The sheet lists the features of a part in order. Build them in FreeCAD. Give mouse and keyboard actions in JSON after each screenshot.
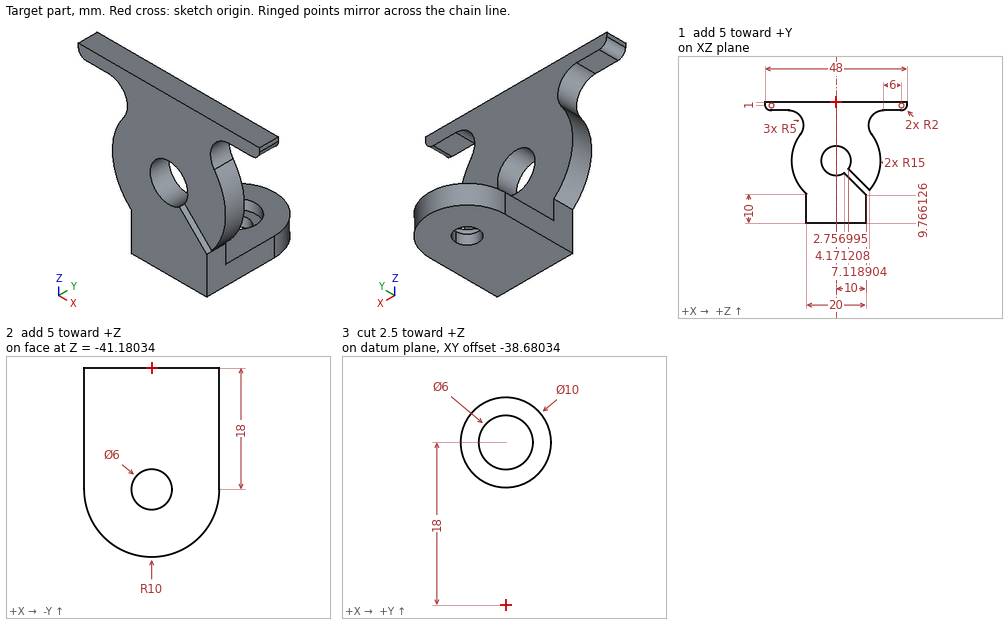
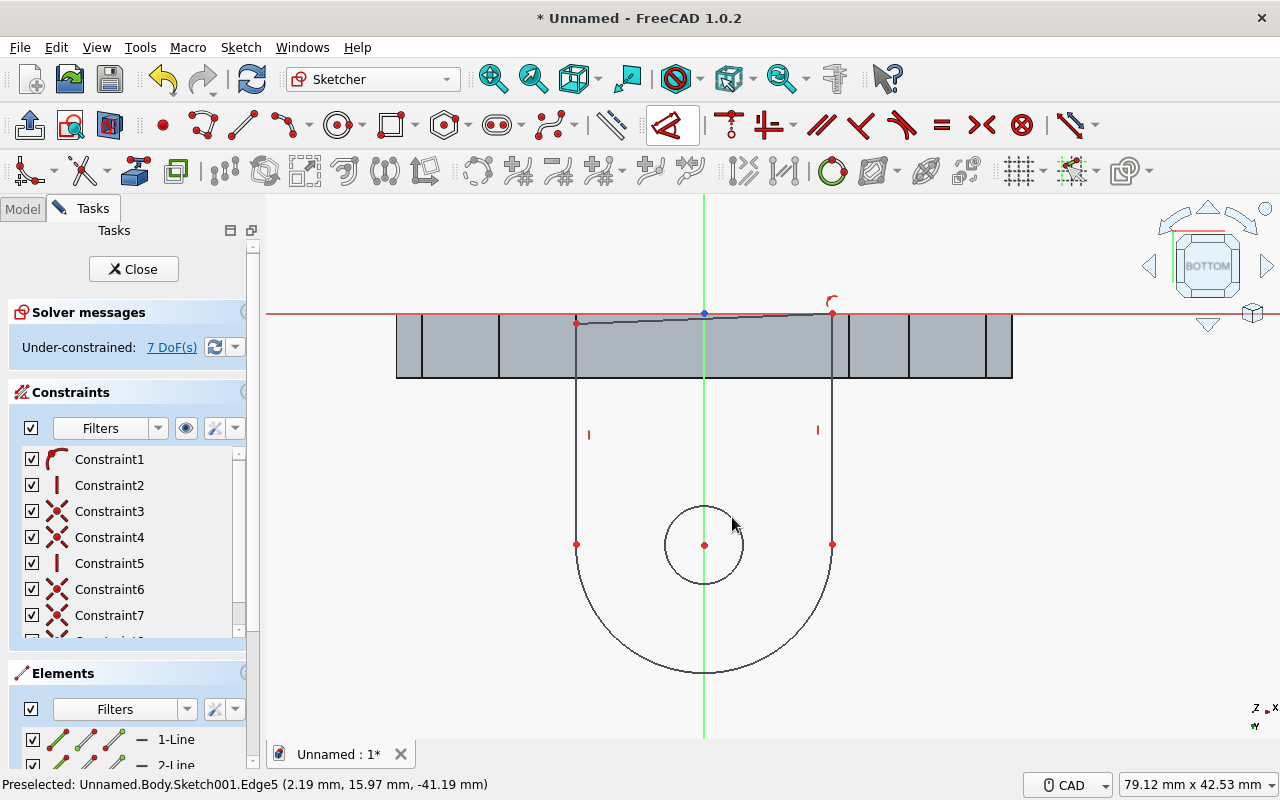
{"action": "left_click", "coordinate": [832, 476]}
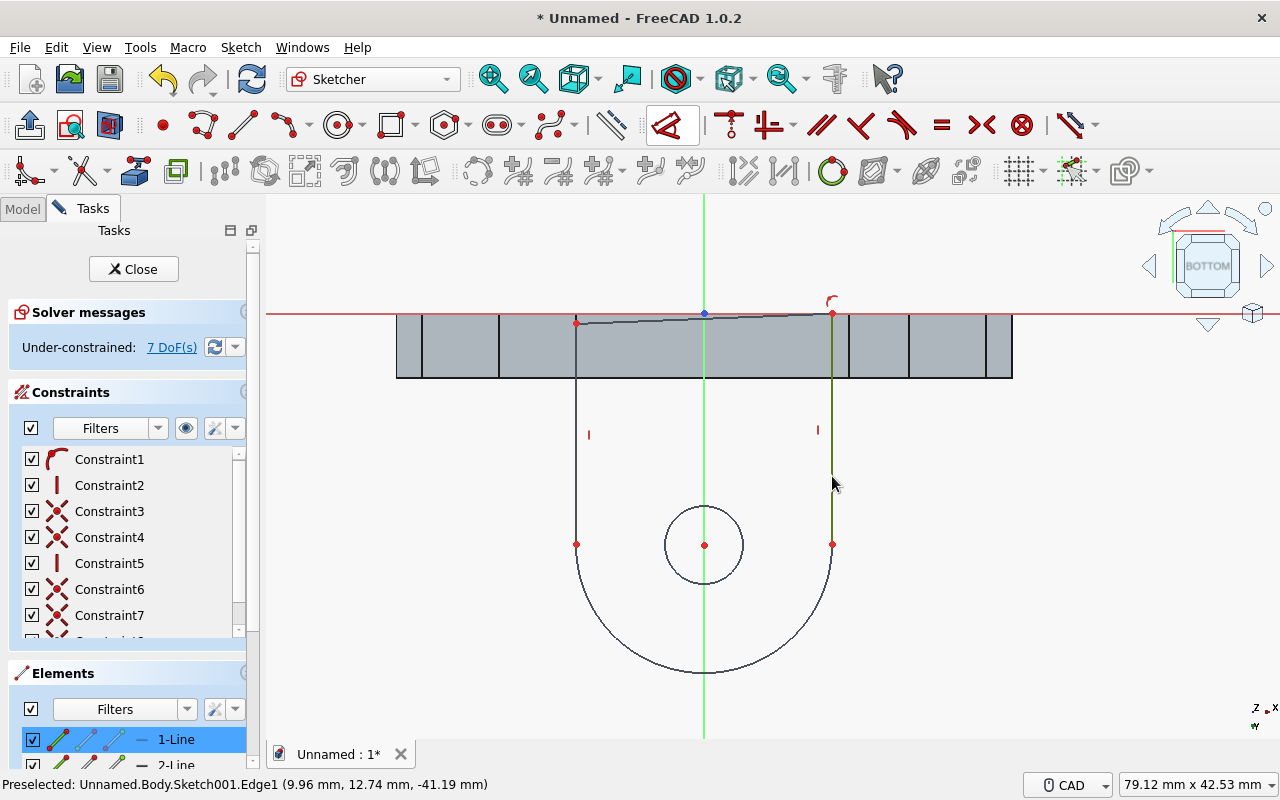
{"action": "left_click", "coordinate": [629, 649]}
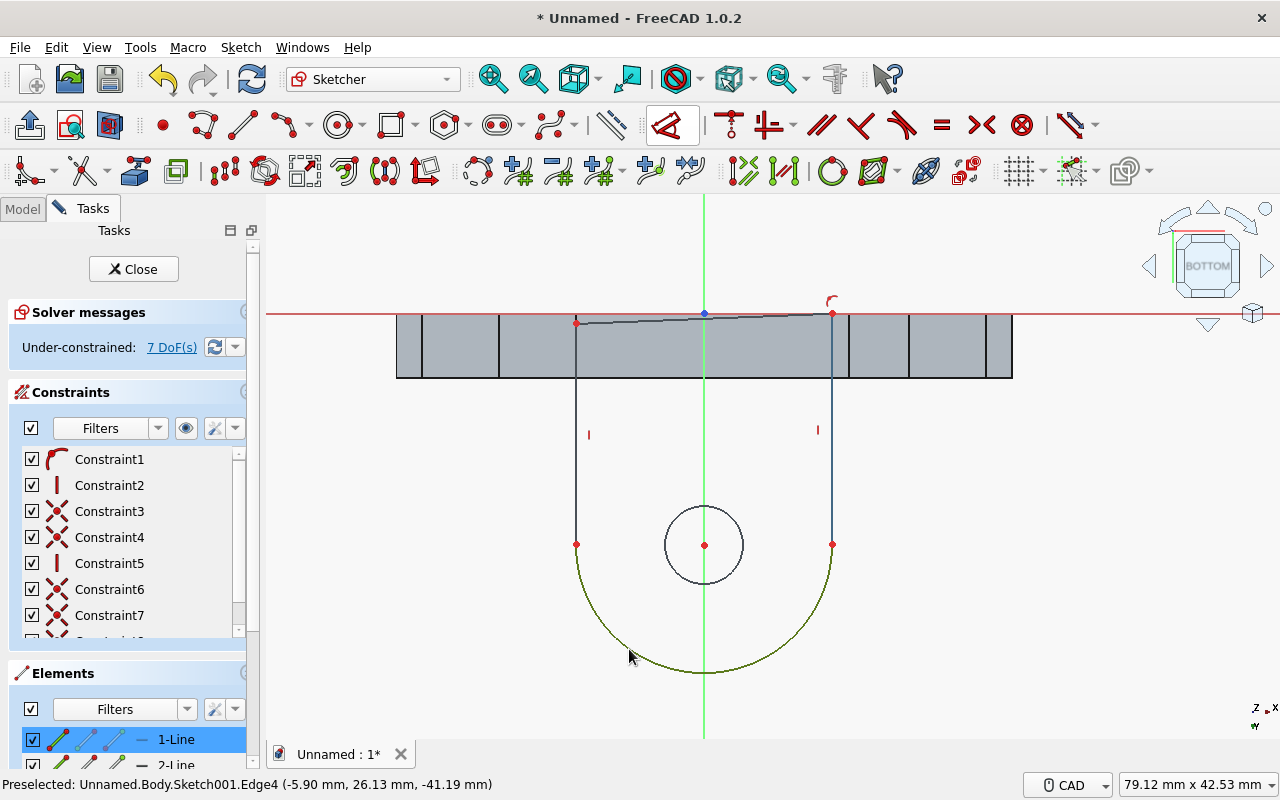
{"action": "key", "text": "t"}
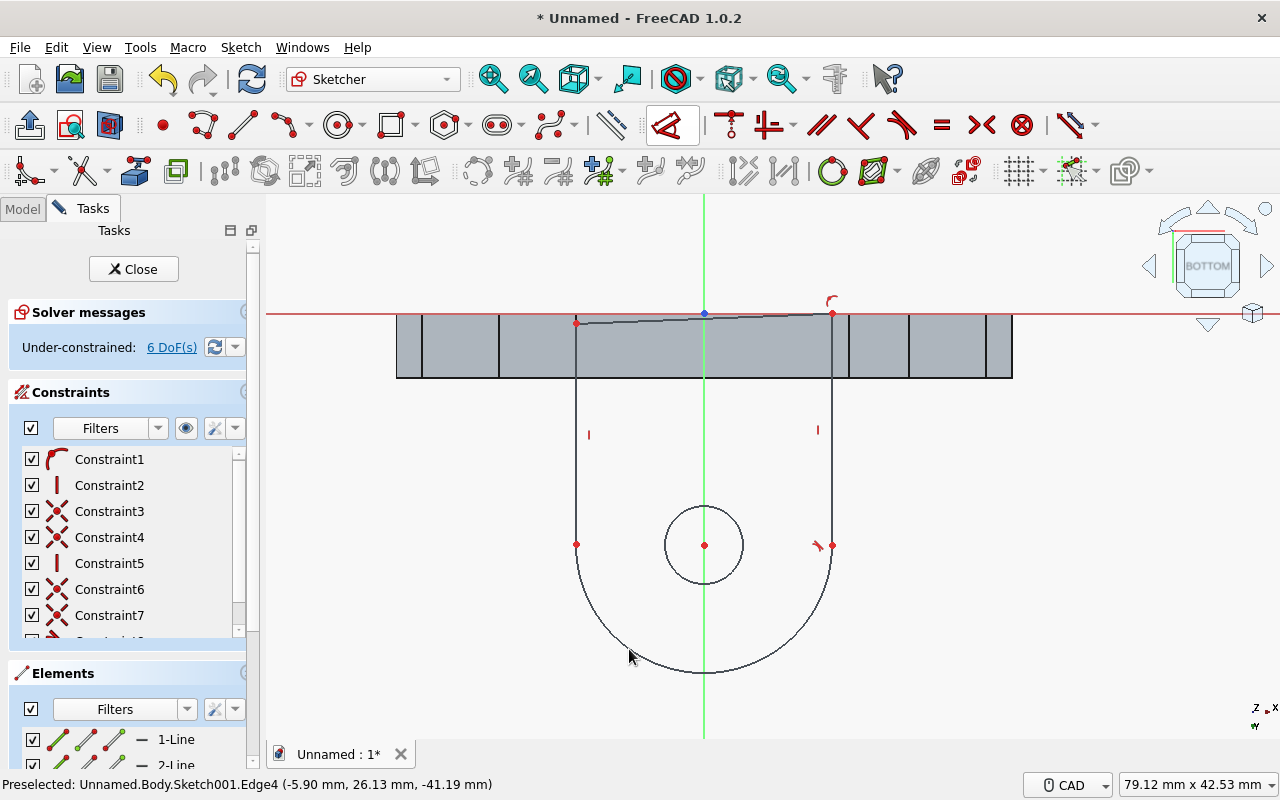
{"action": "left_click", "coordinate": [576, 390]}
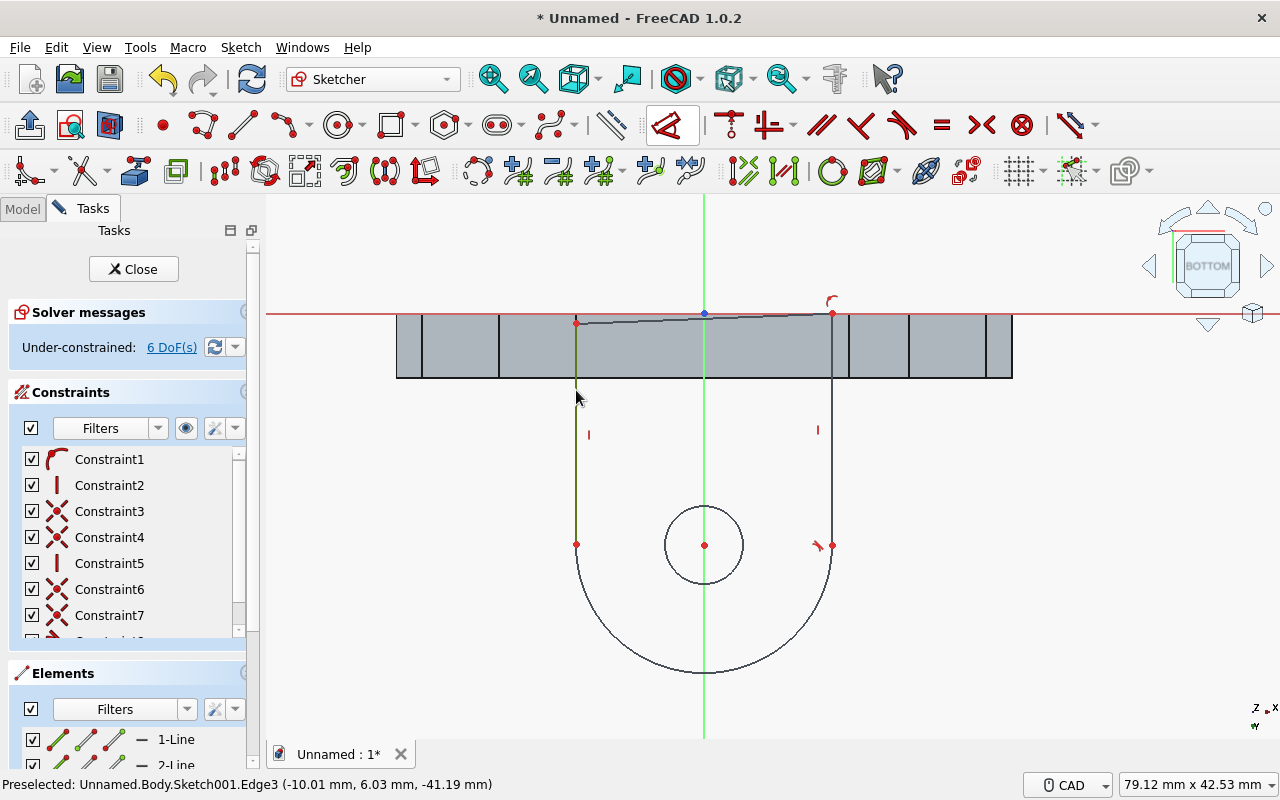
{"action": "left_click", "coordinate": [629, 649]}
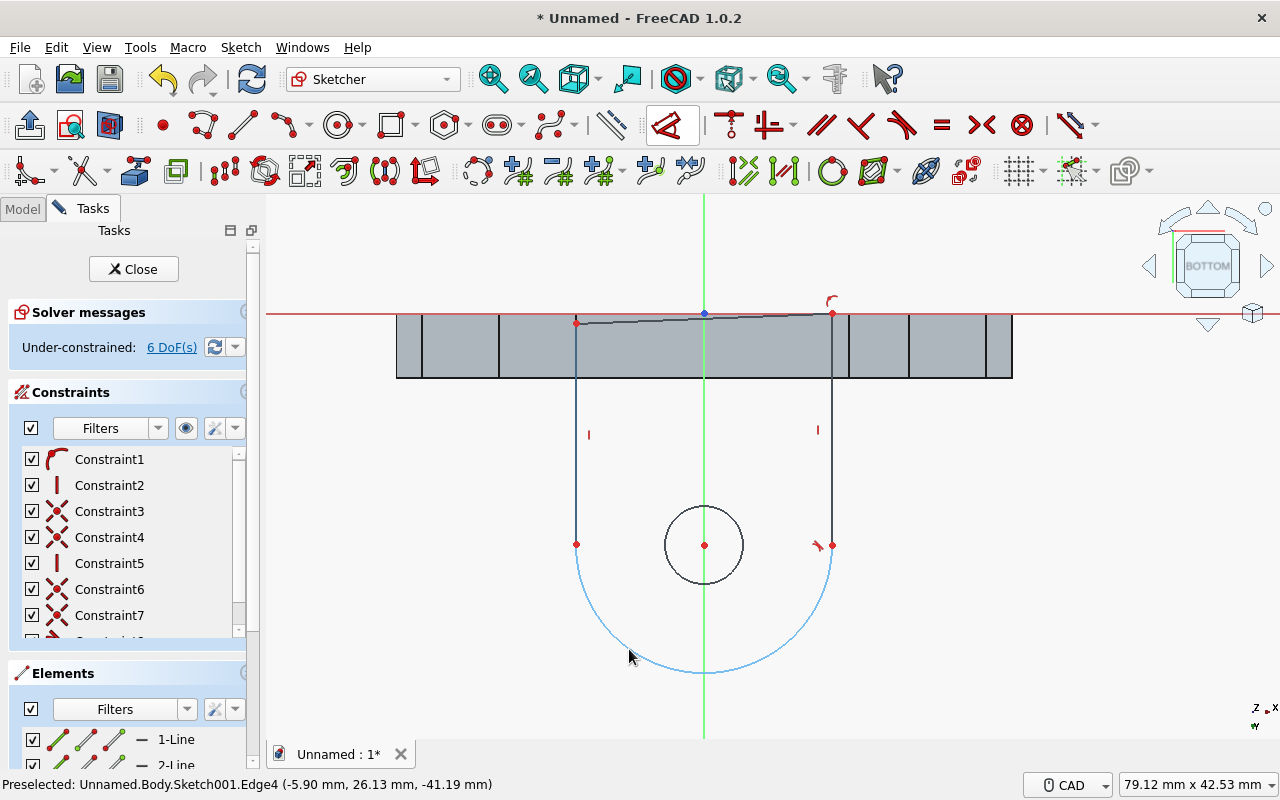
{"action": "key", "text": "t"}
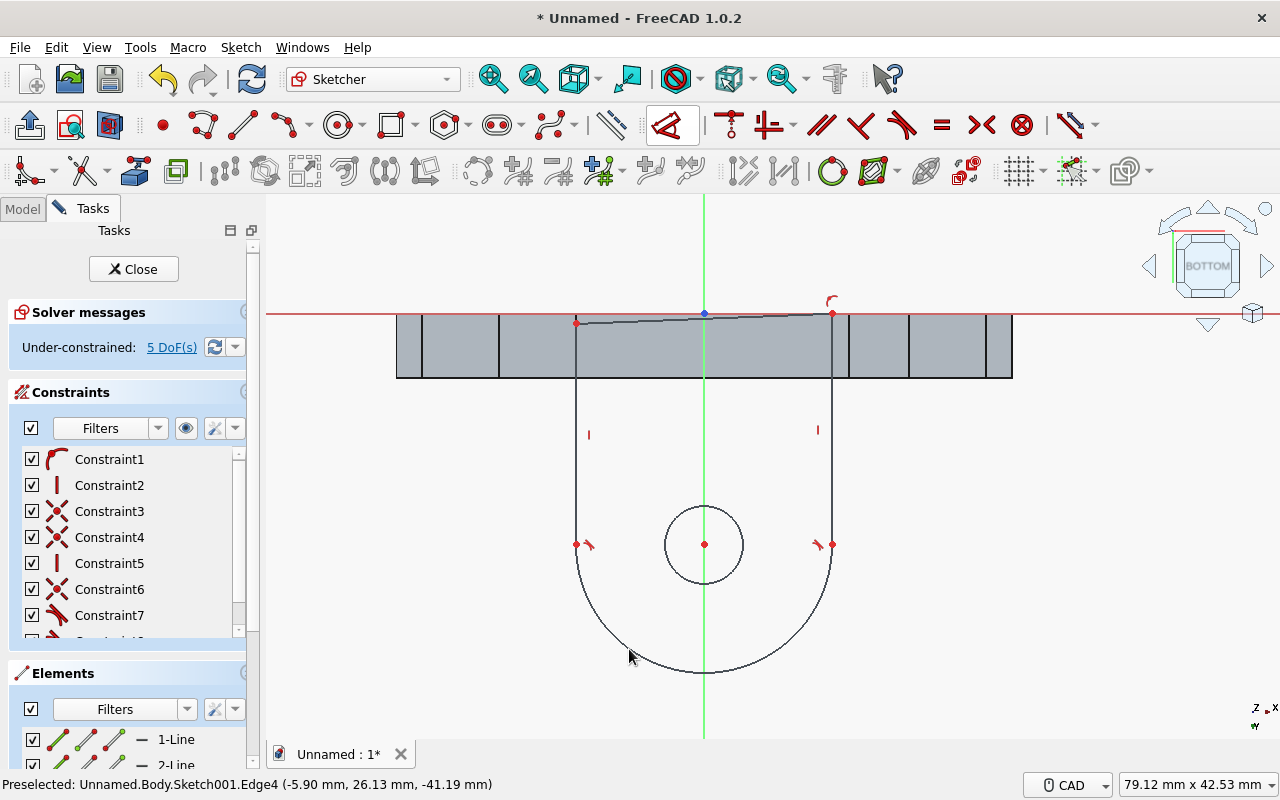
{"action": "left_click", "coordinate": [755, 317]}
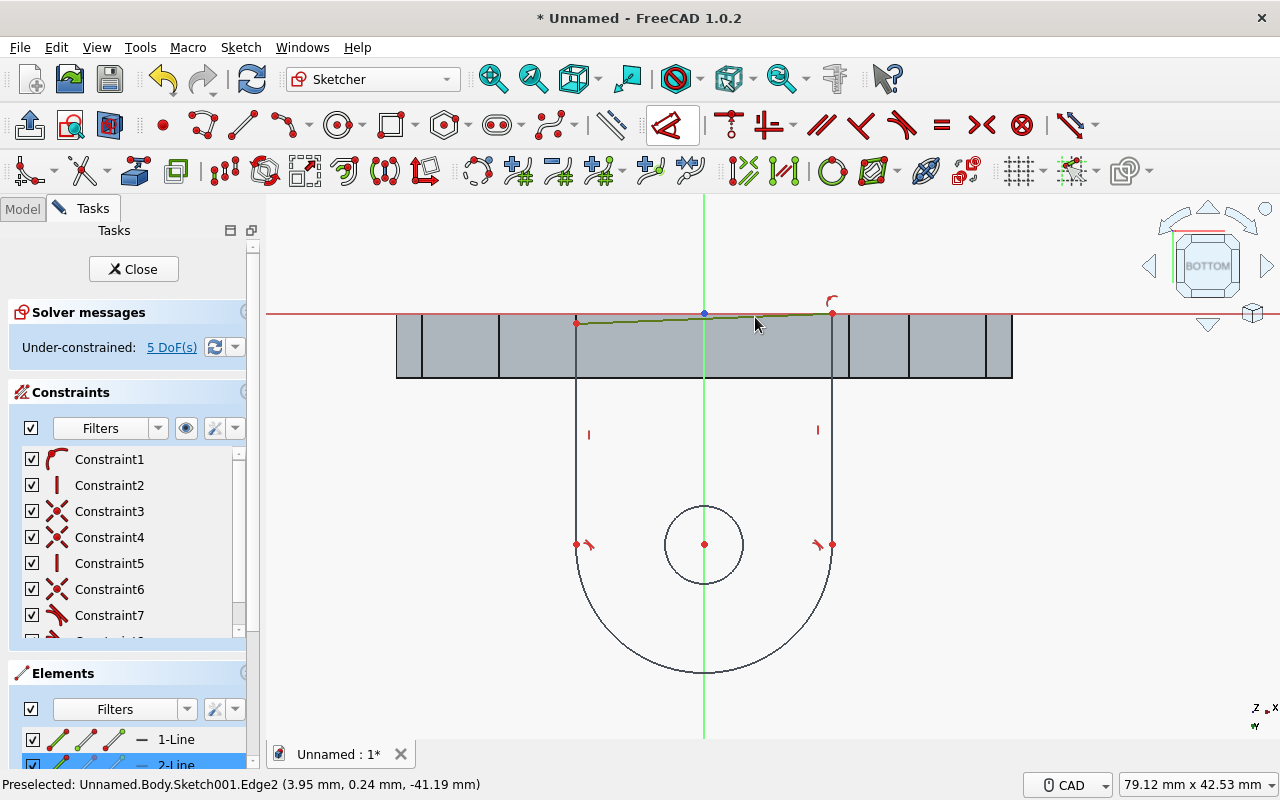
{"action": "left_click", "coordinate": [796, 126]}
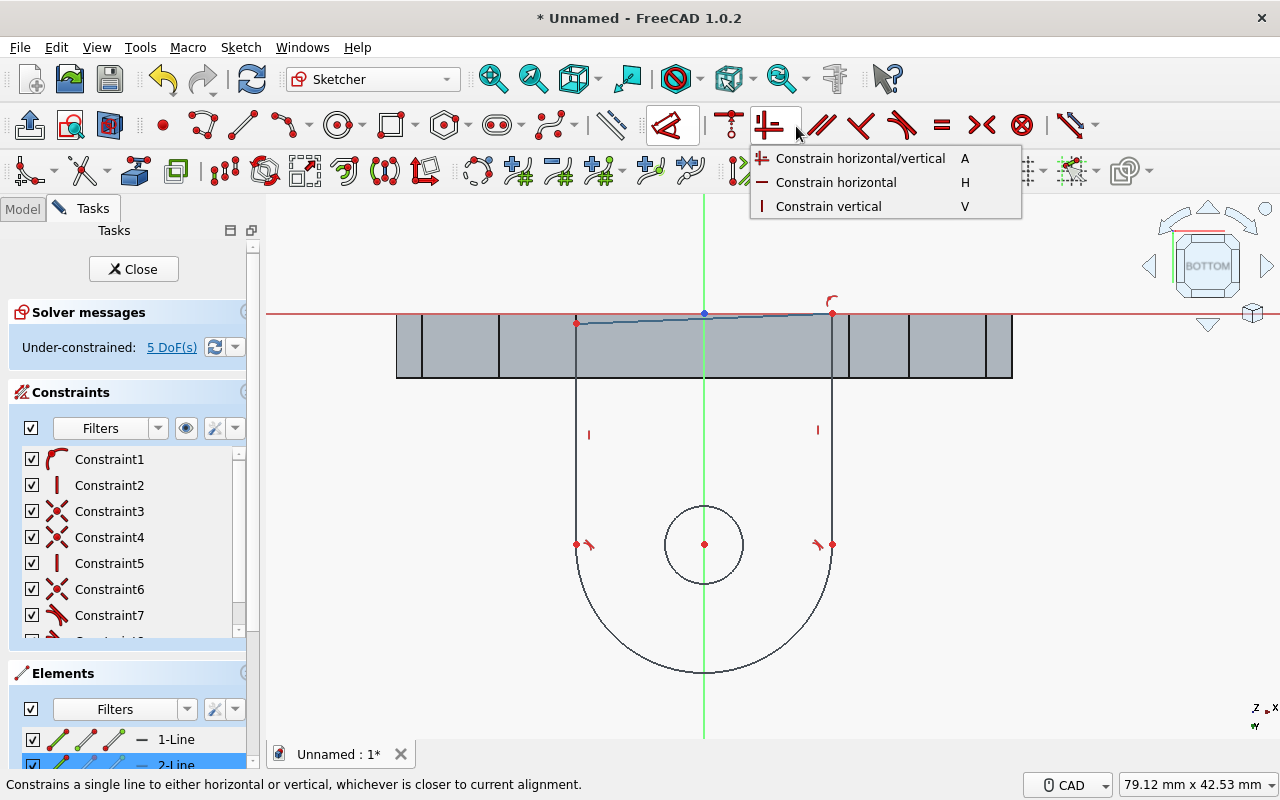
{"action": "left_click", "coordinate": [886, 182]}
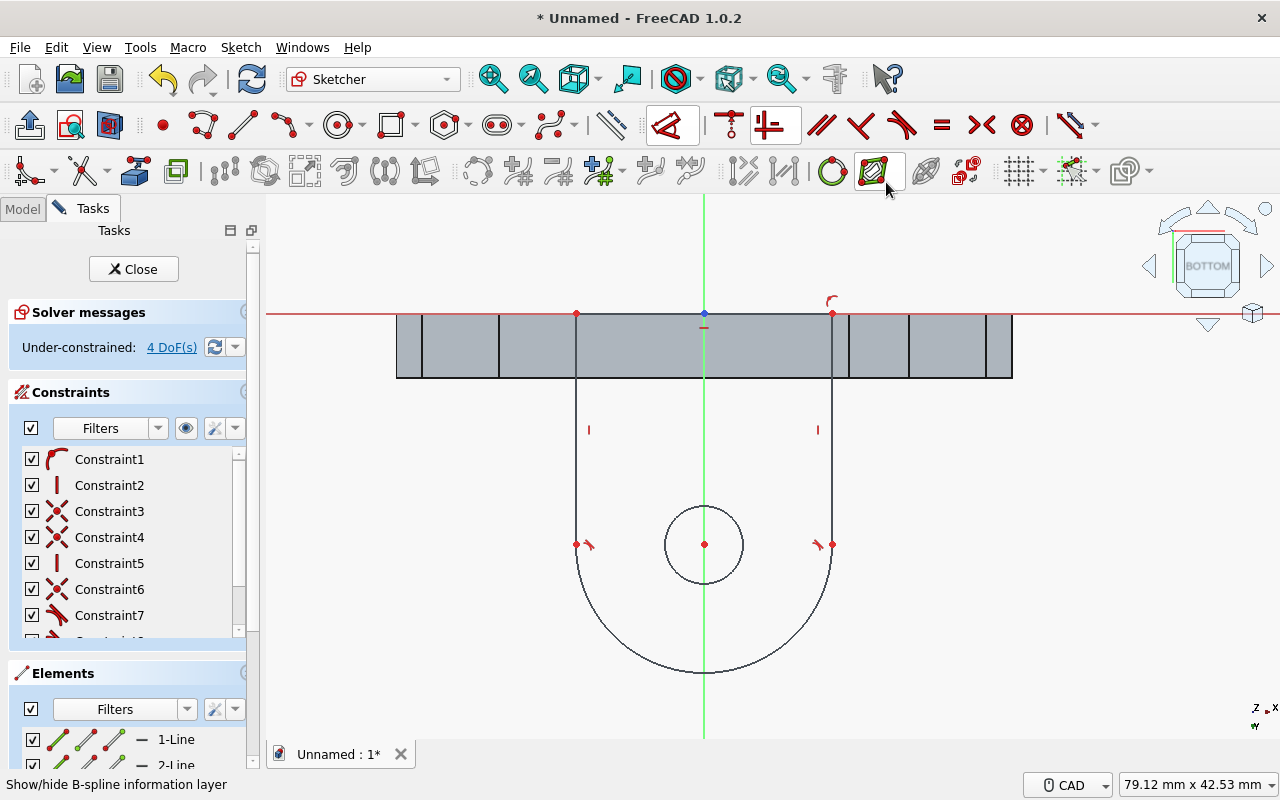
{"action": "left_click", "coordinate": [704, 545]}